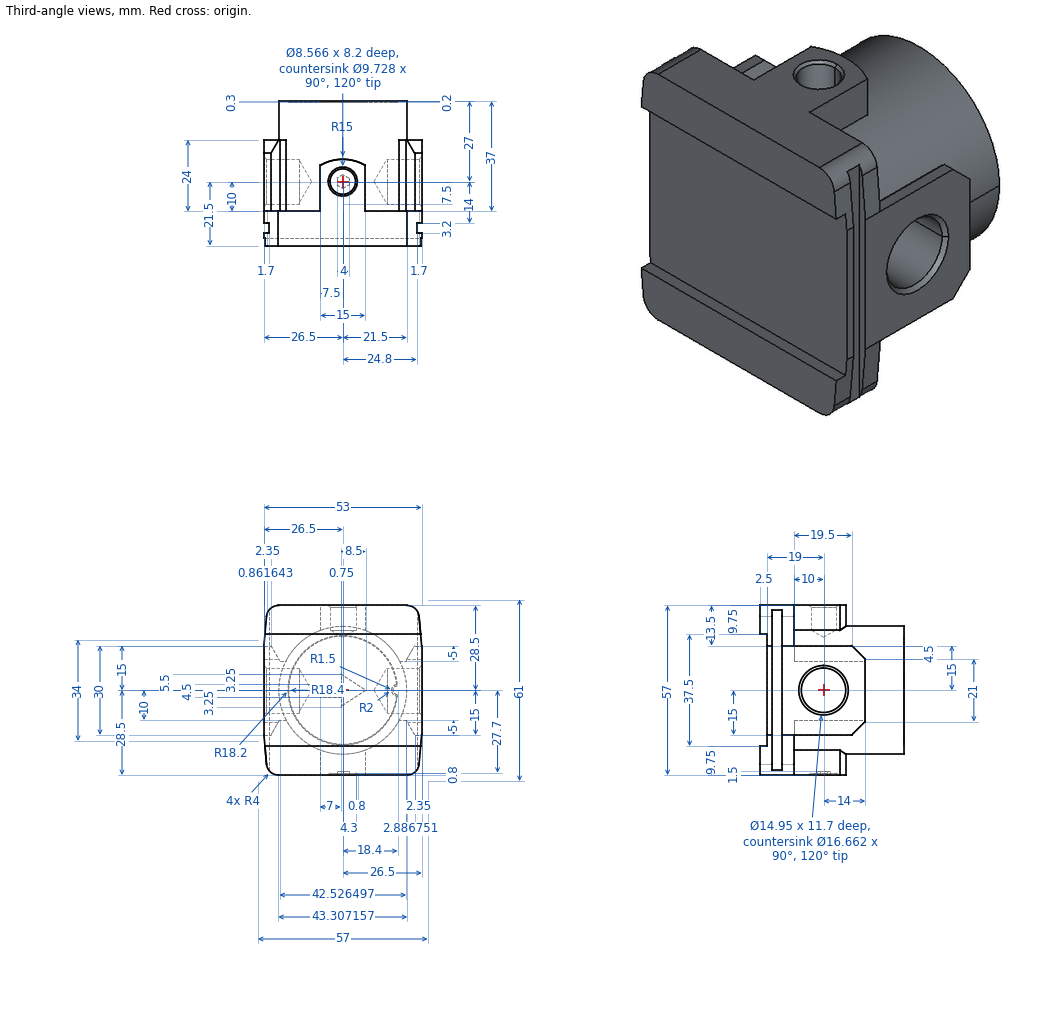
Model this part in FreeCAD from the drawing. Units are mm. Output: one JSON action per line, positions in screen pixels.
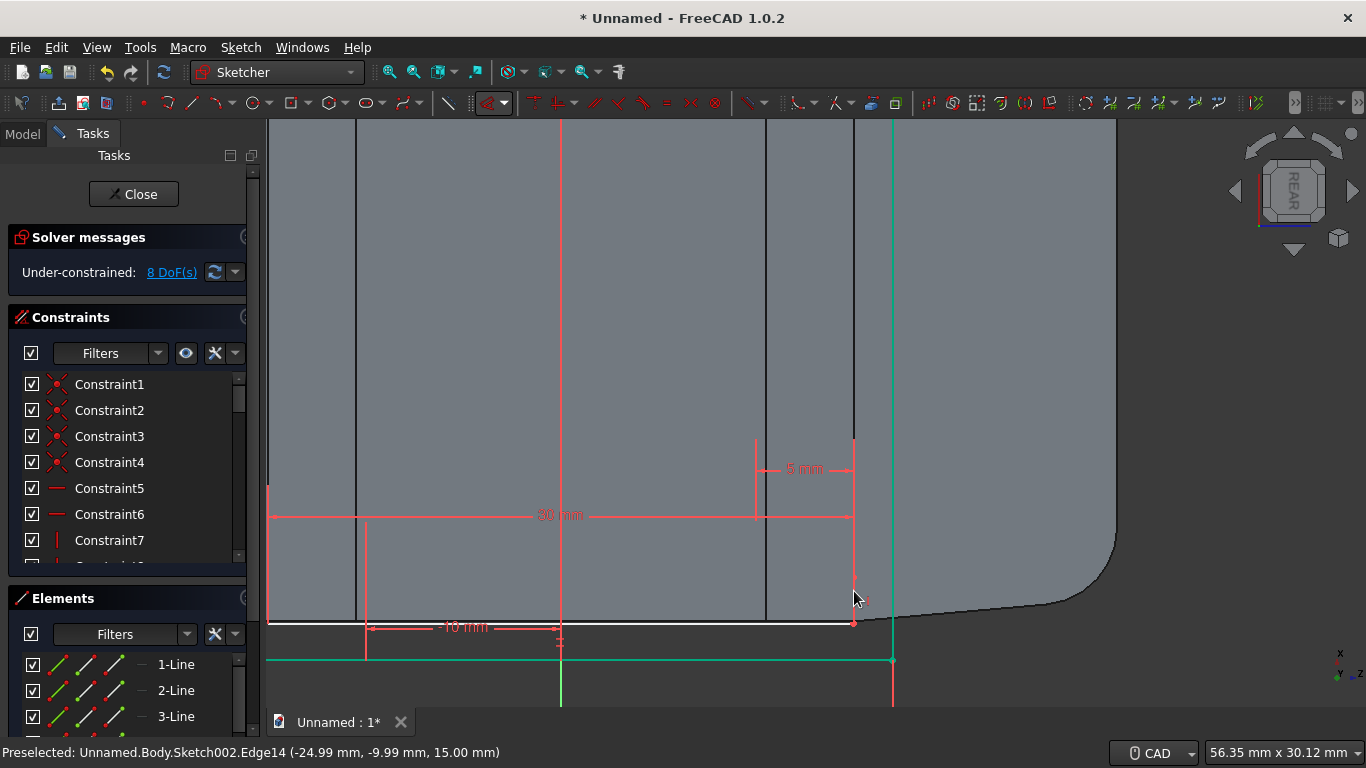
{"action": "key", "text": "i"}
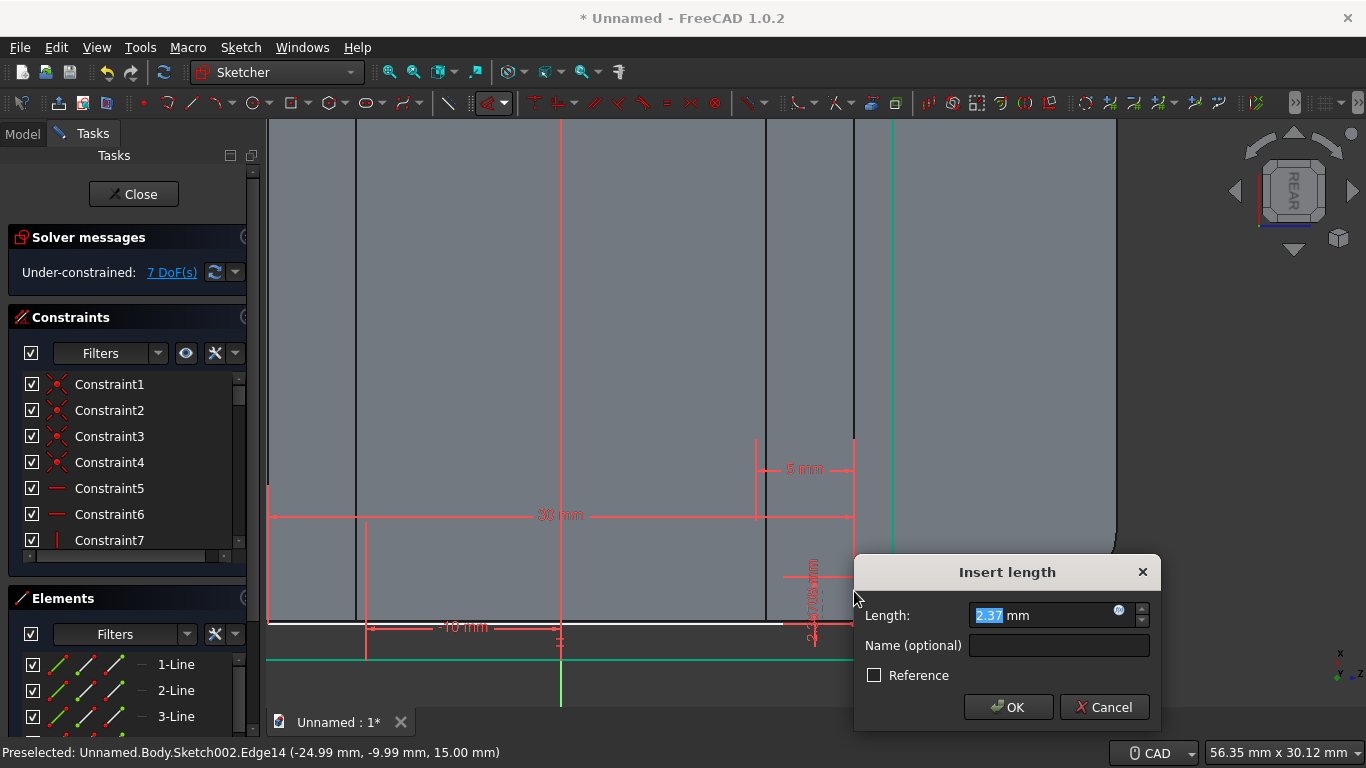
{"action": "type", "text": "2.35"}
{"action": "key", "text": "Return"}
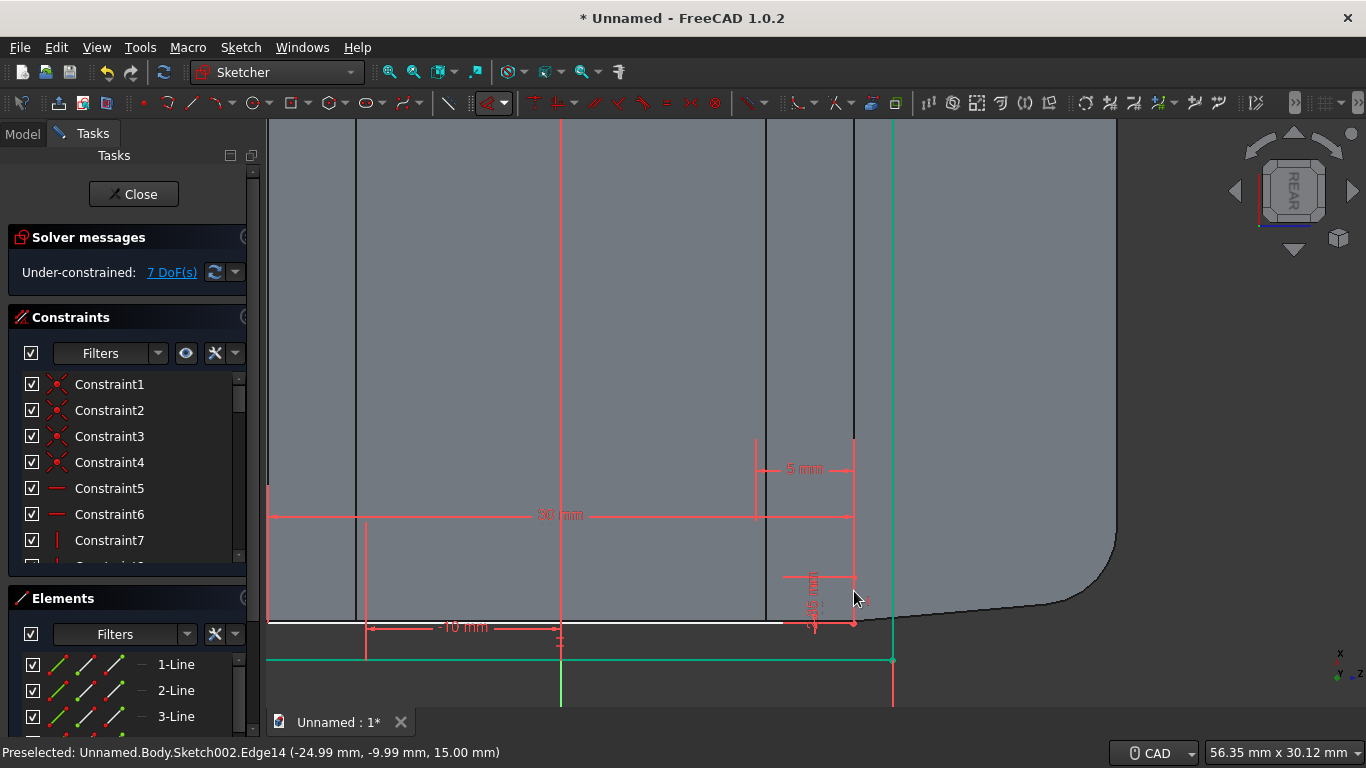
{"action": "scroll", "coordinate": [856, 593], "scroll_direction": "down", "scroll_amount": 5}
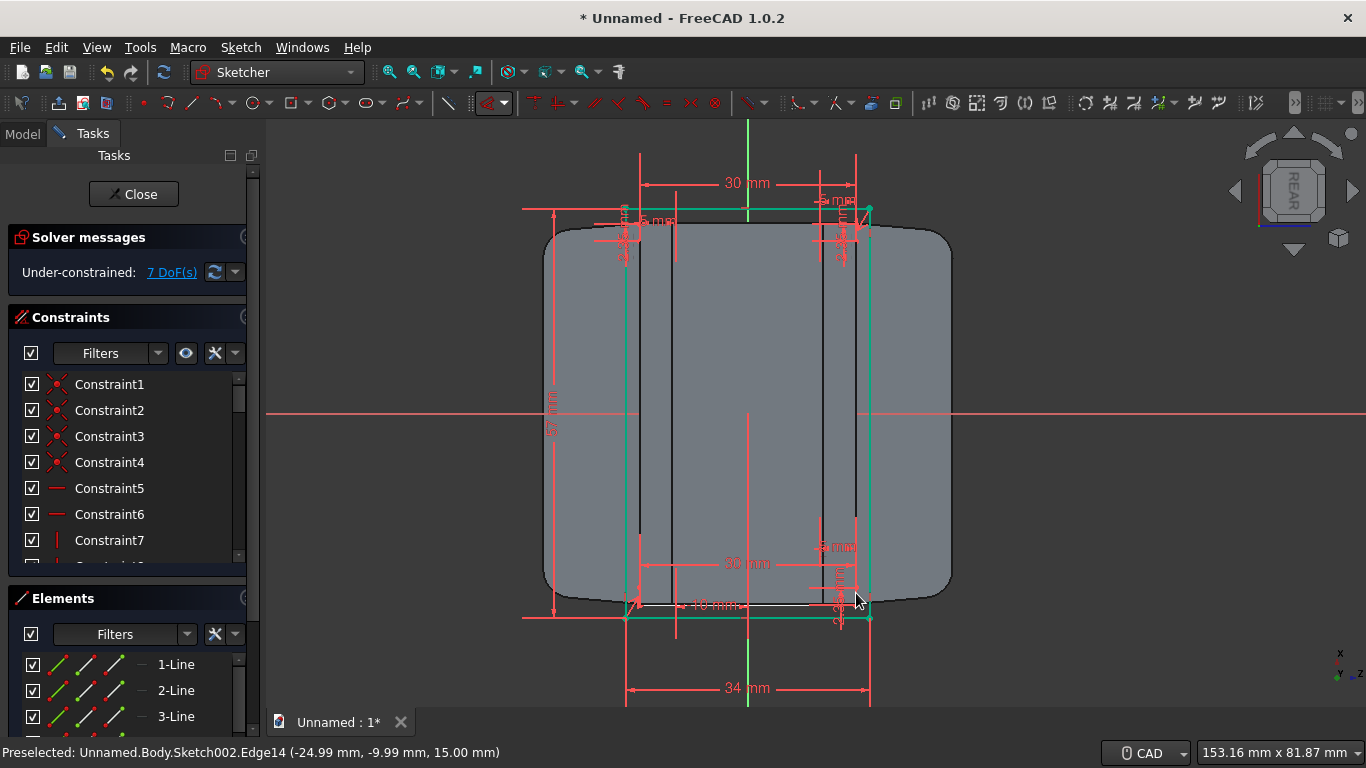
{"action": "scroll", "coordinate": [640, 600], "scroll_direction": "up", "scroll_amount": 6}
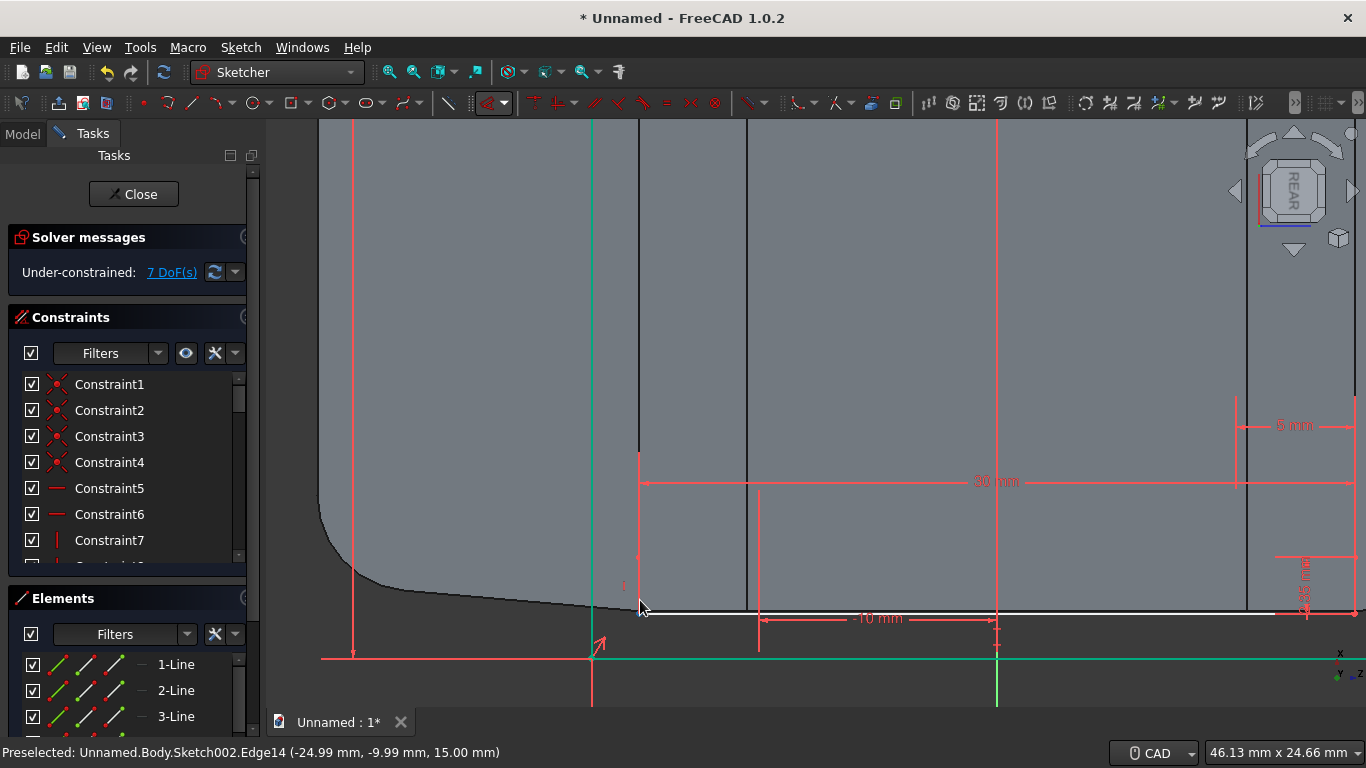
{"action": "left_click", "coordinate": [639, 597]}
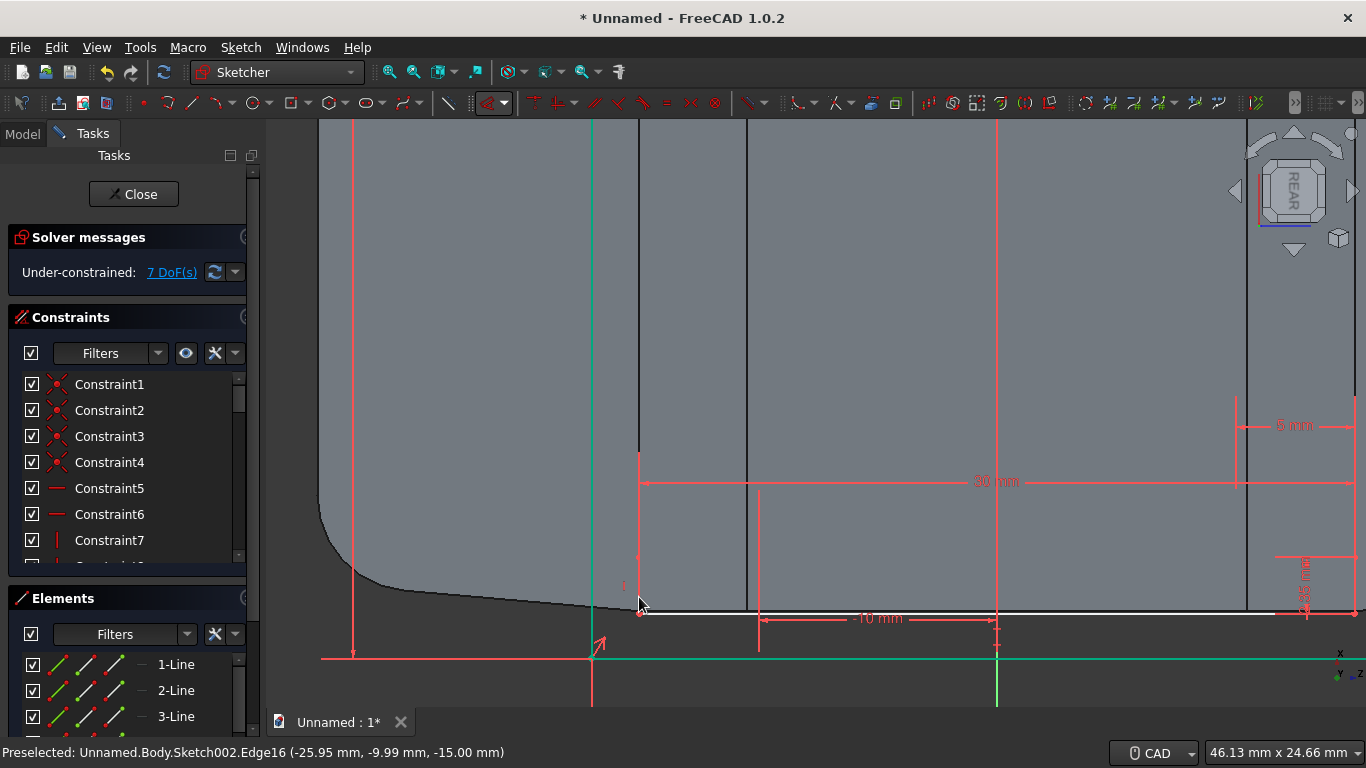
{"action": "key", "text": "i"}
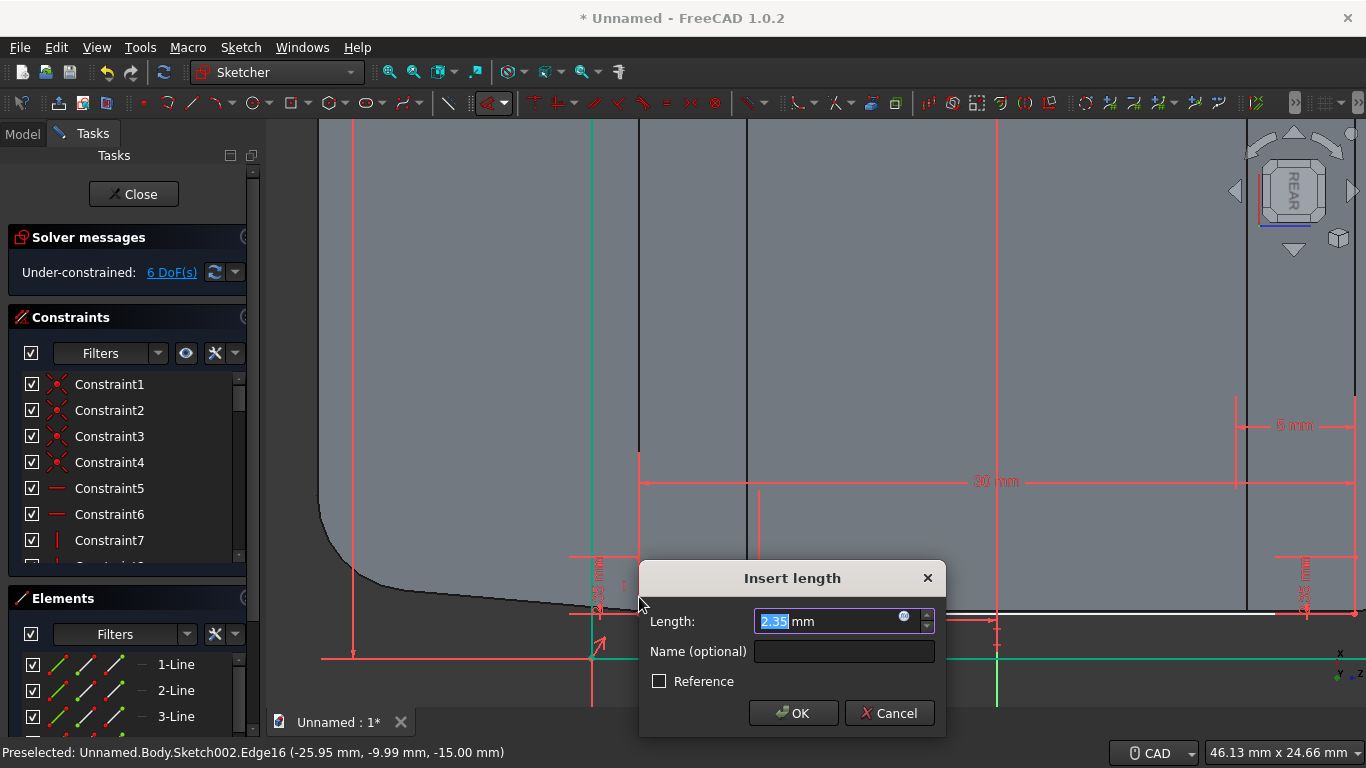
{"action": "type", "text": "2.35"}
{"action": "key", "text": "Return"}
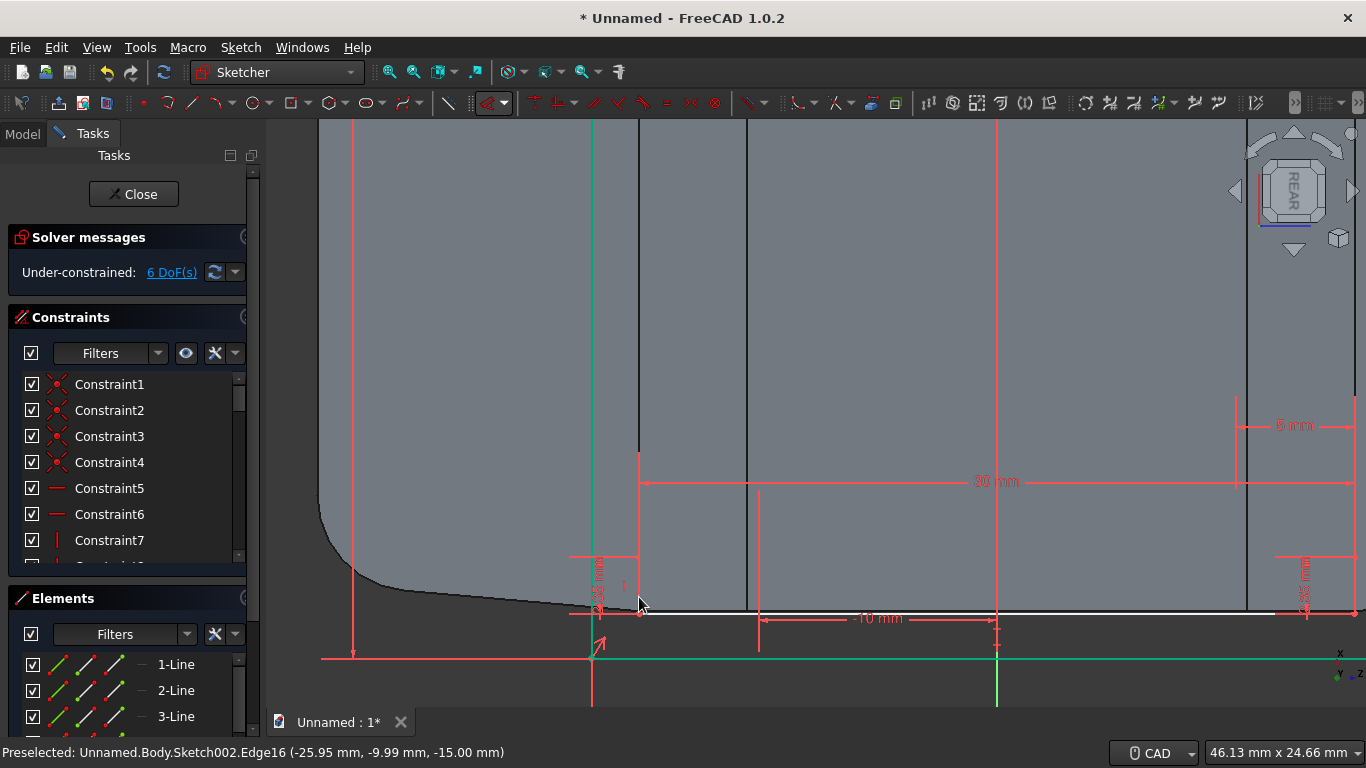
{"action": "scroll", "coordinate": [640, 600], "scroll_direction": "down", "scroll_amount": 6}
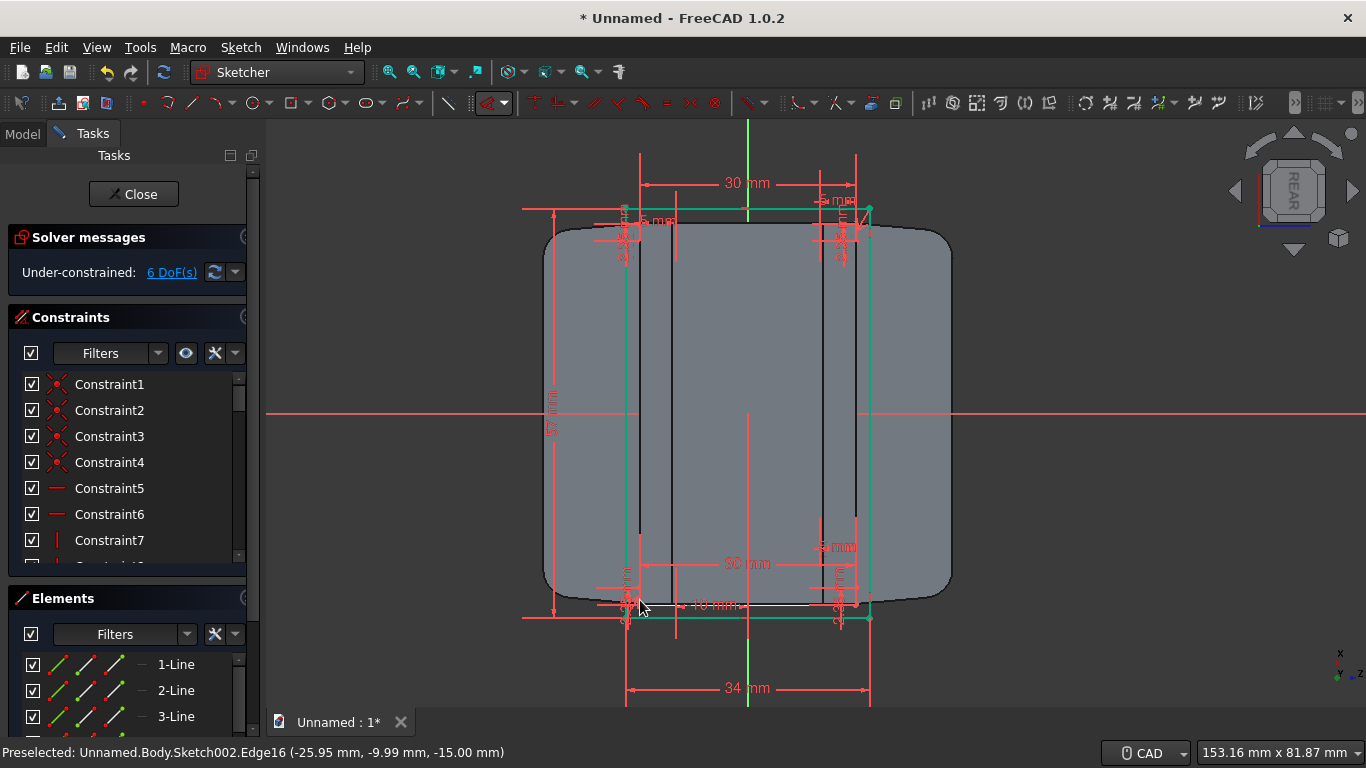
{"action": "left_click", "coordinate": [640, 224]}